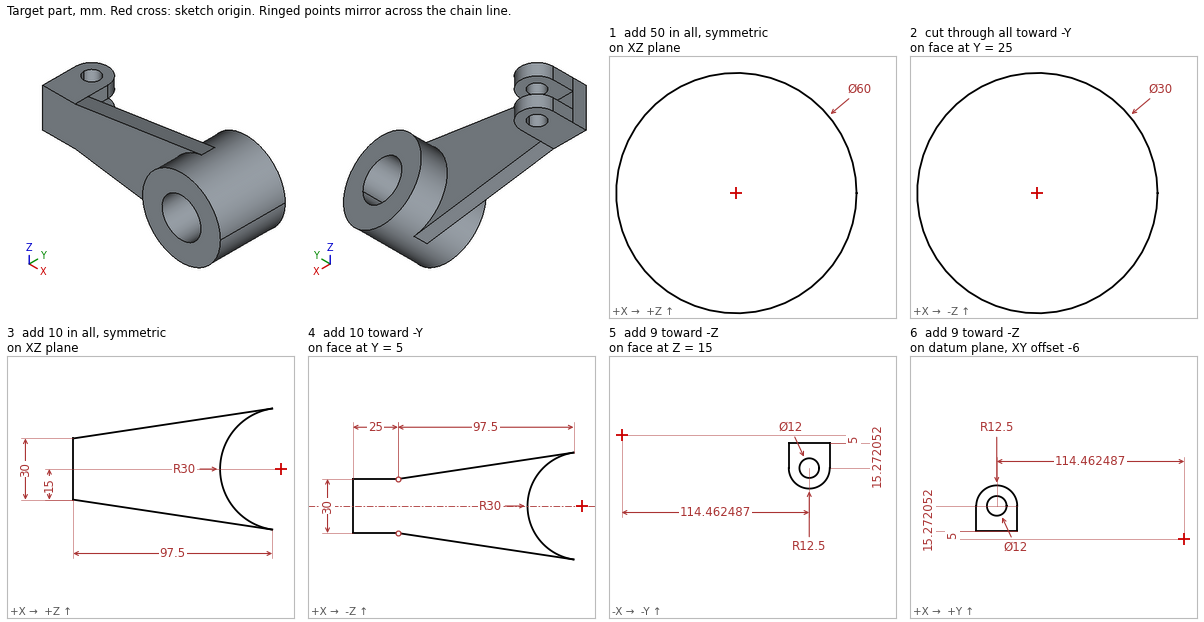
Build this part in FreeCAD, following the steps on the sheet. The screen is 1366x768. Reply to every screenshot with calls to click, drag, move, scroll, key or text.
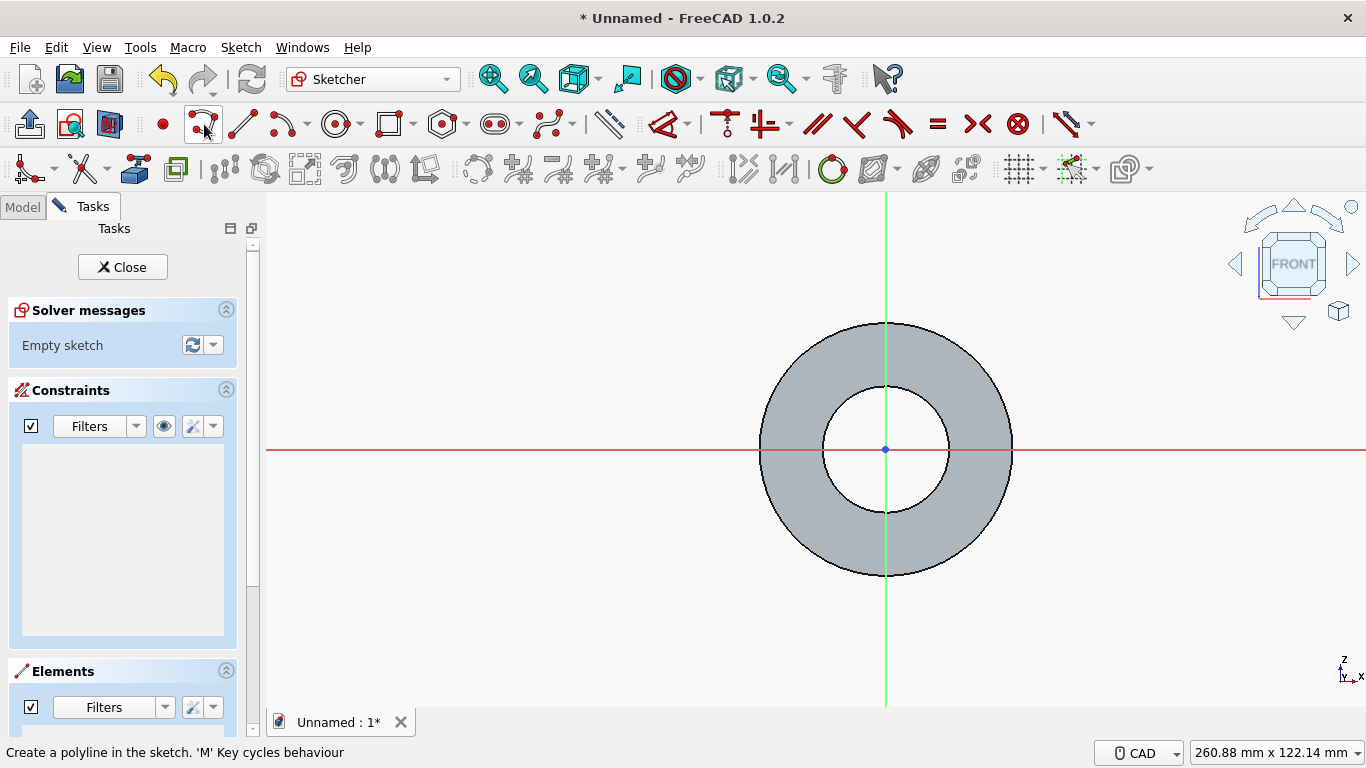
click(867, 575)
click(456, 513)
click(456, 386)
click(867, 324)
right_click(867, 324)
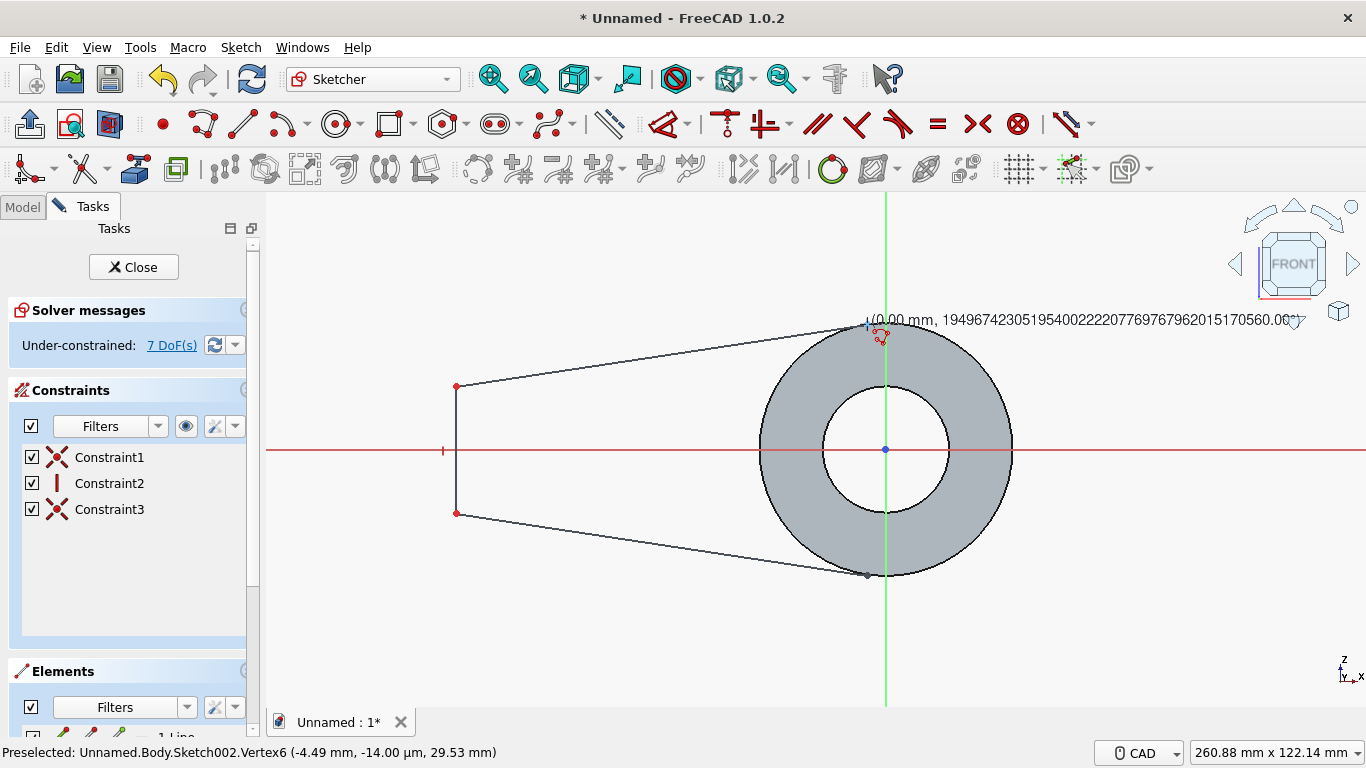
click(310, 124)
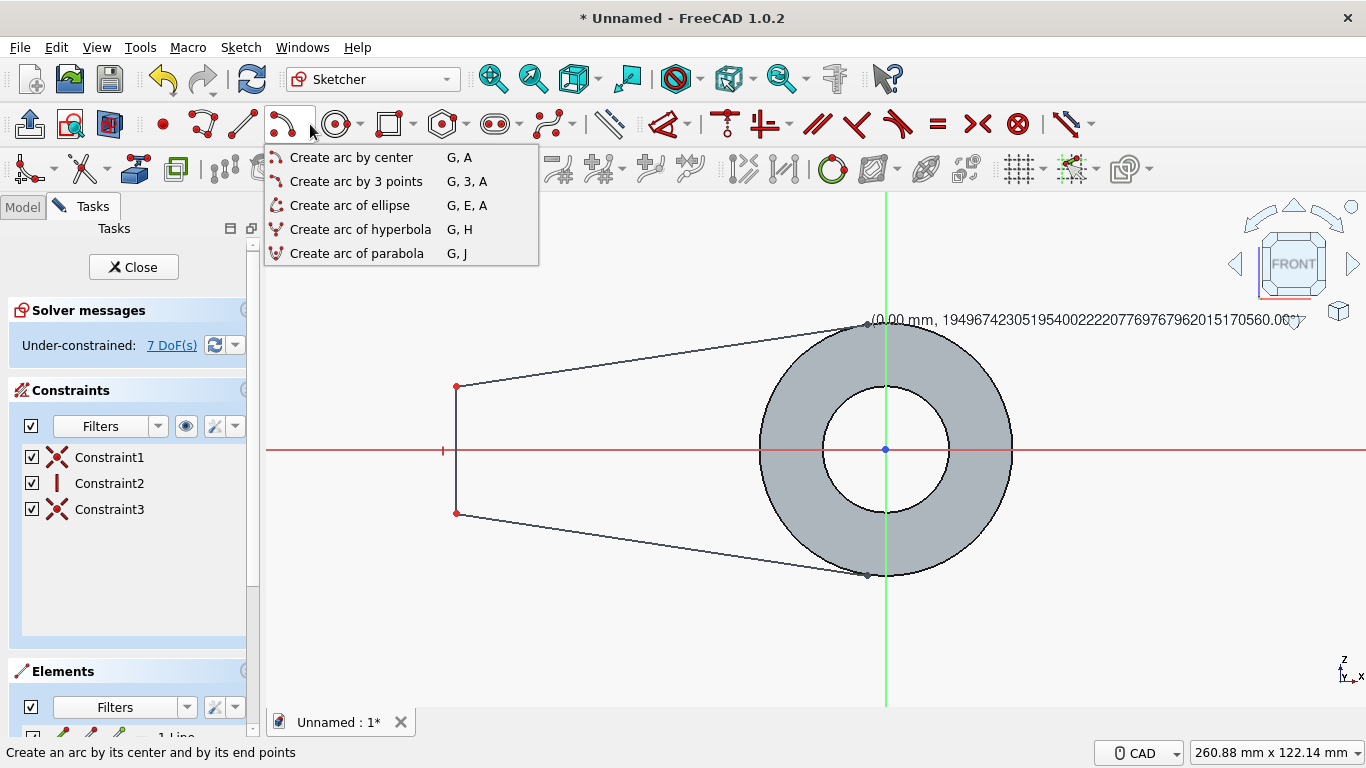
click(402, 181)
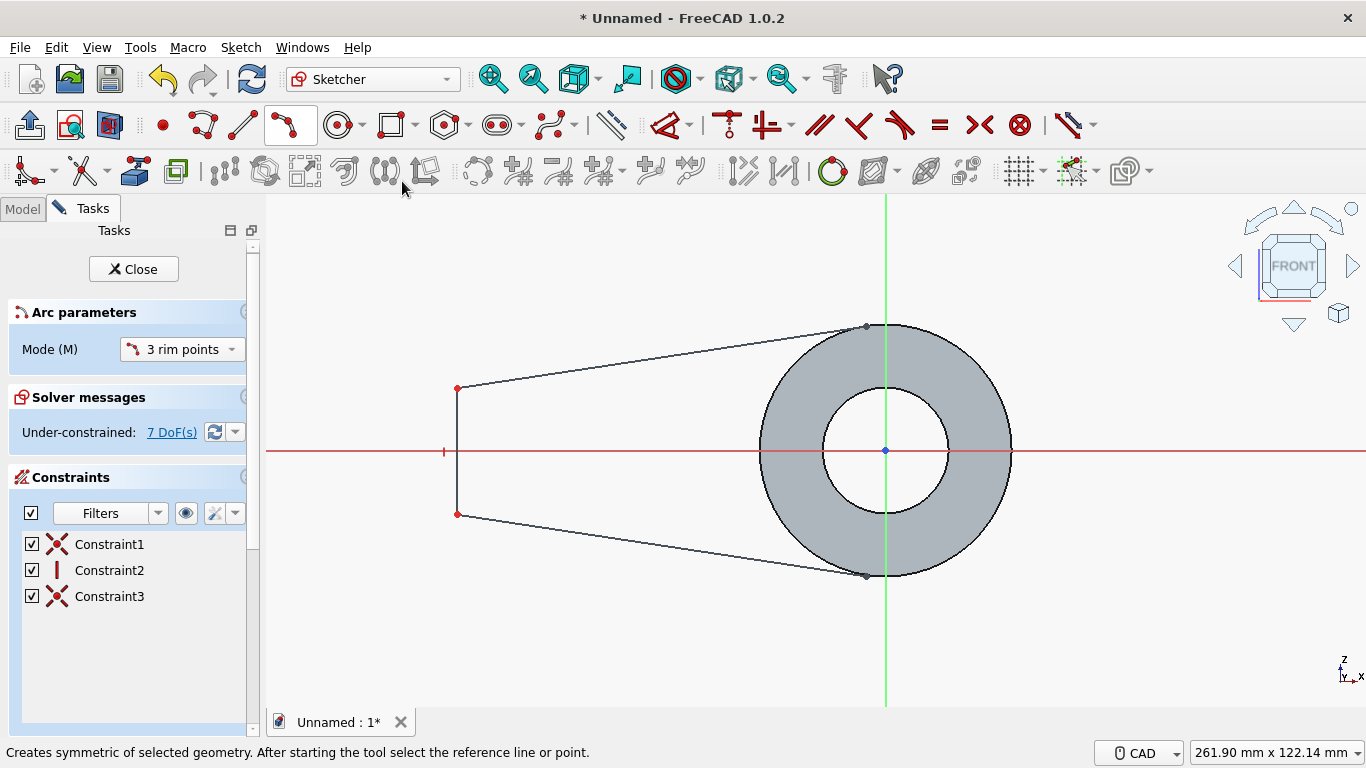
click(867, 326)
click(867, 577)
click(765, 415)
key(Escape)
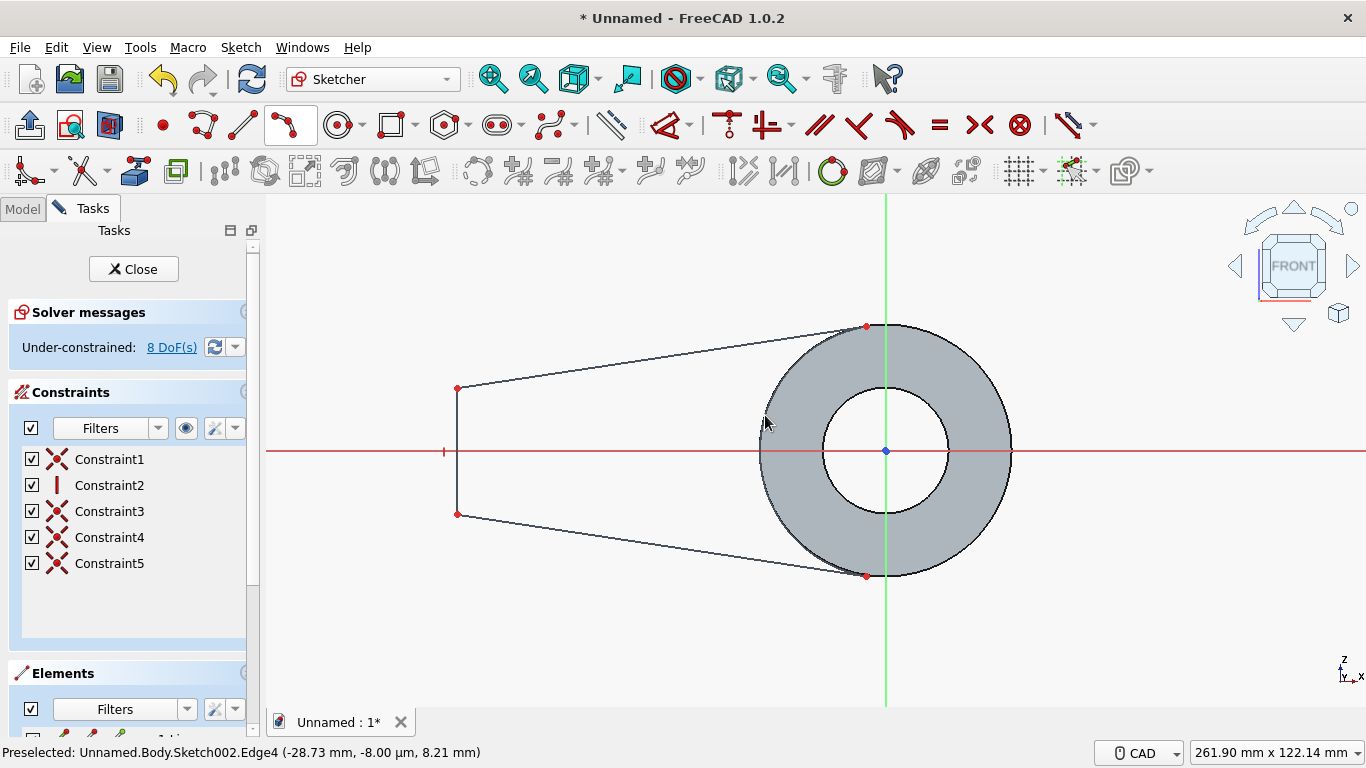
click(744, 558)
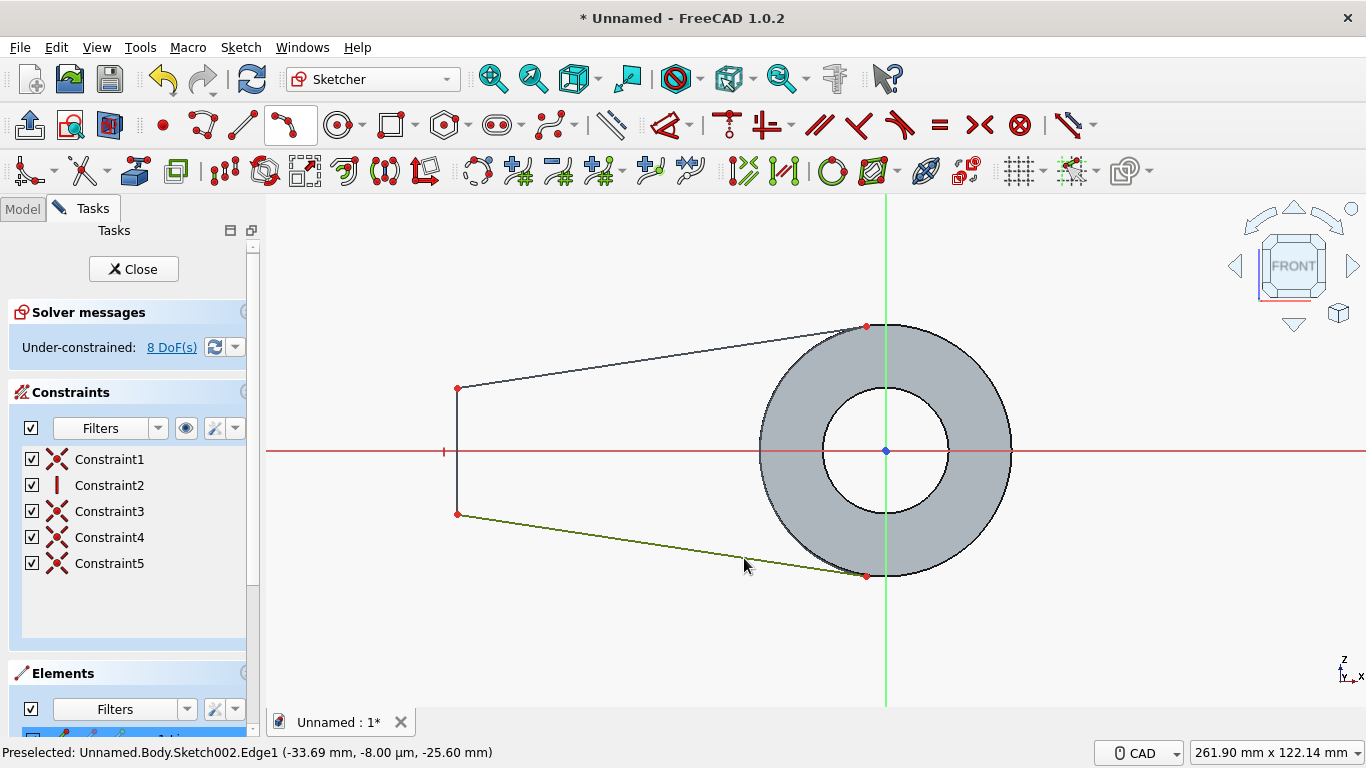
click(780, 384)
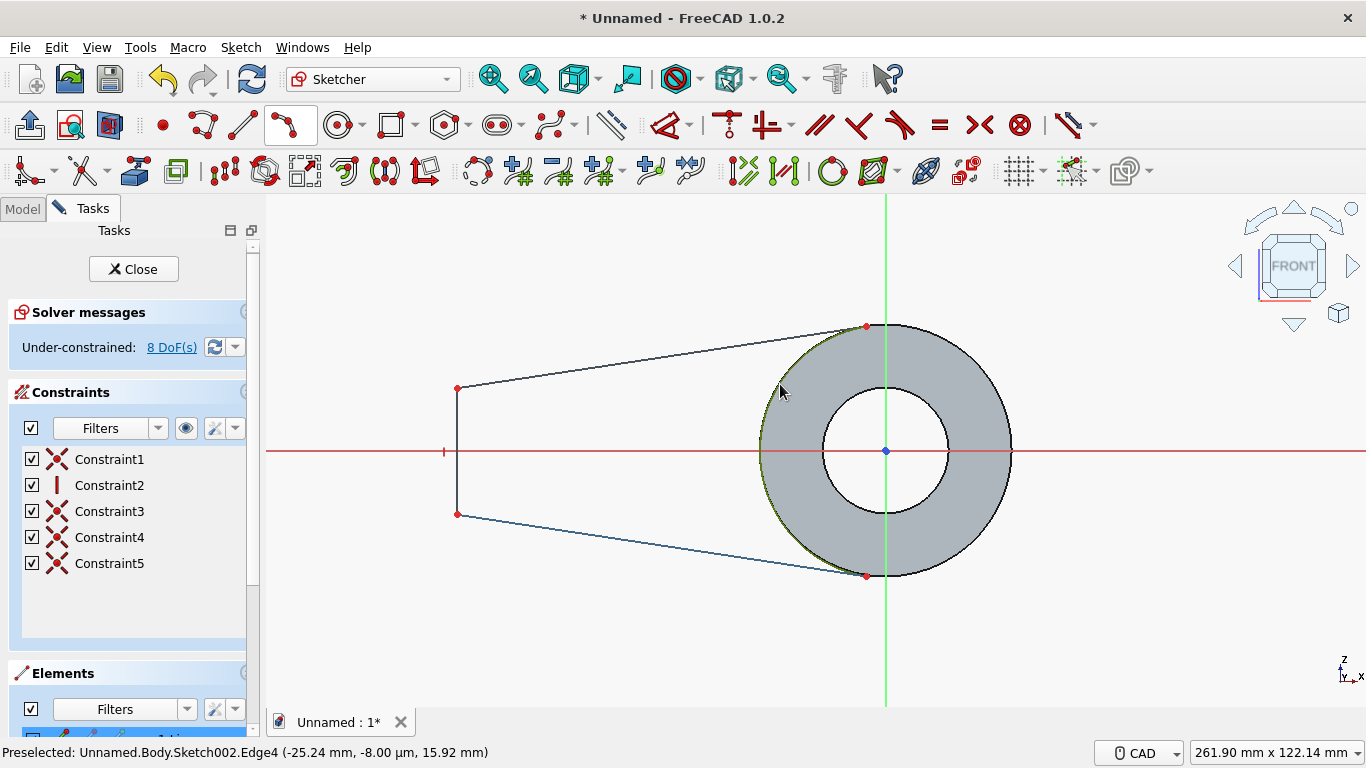
click(900, 126)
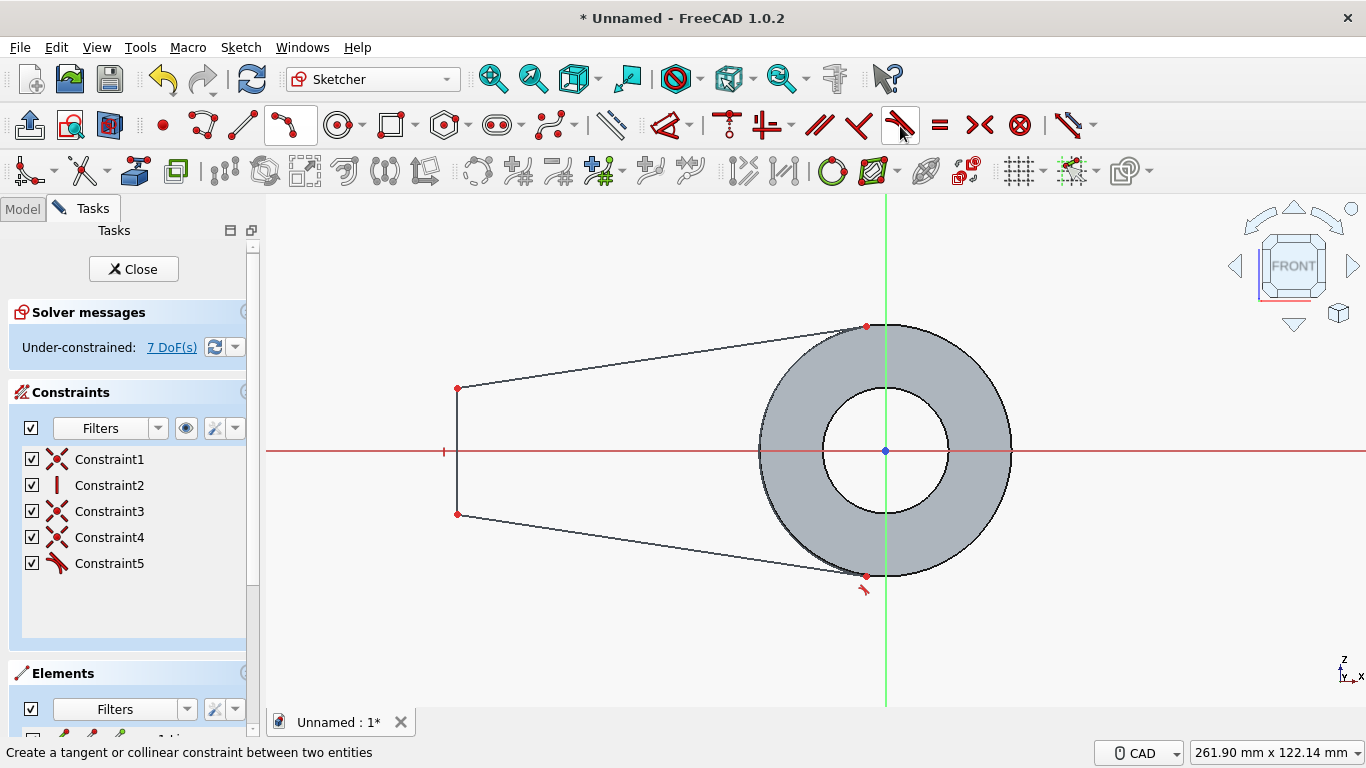
click(580, 370)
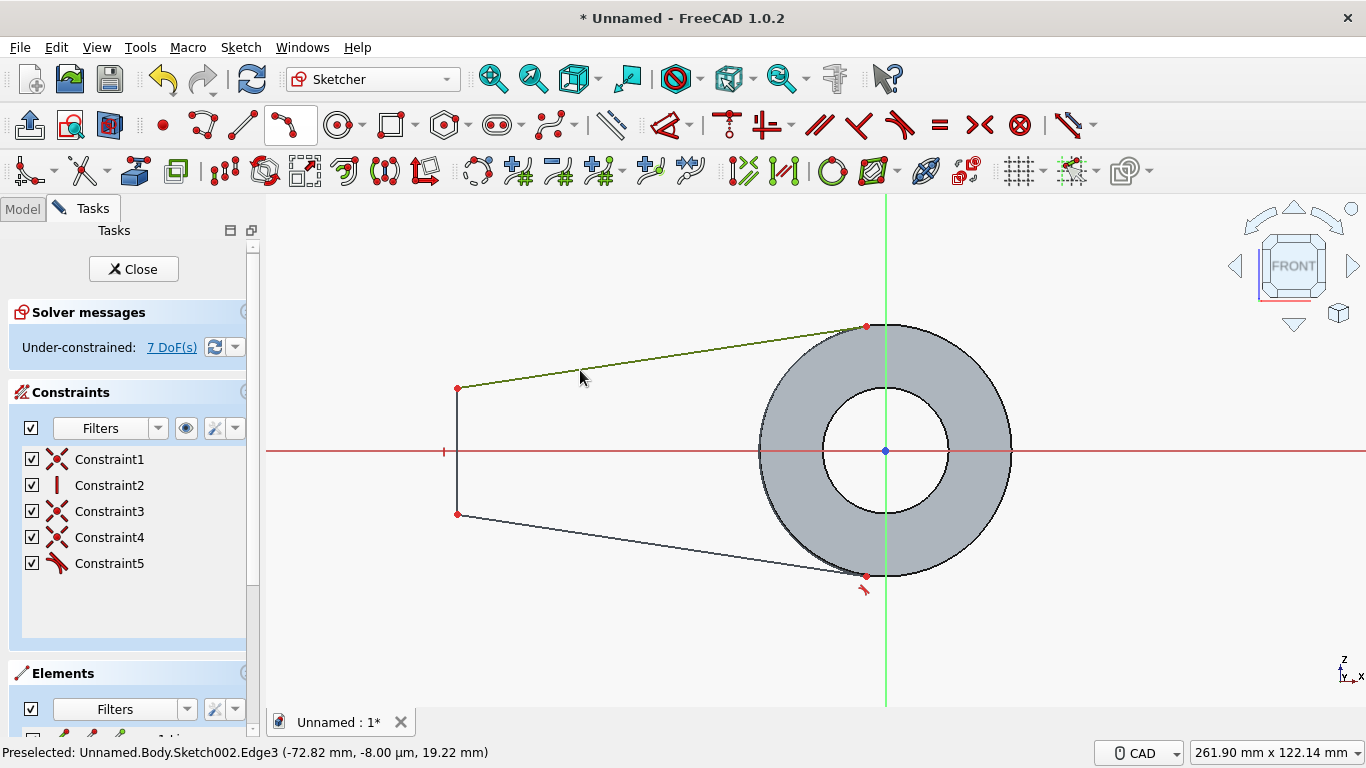
click(779, 383)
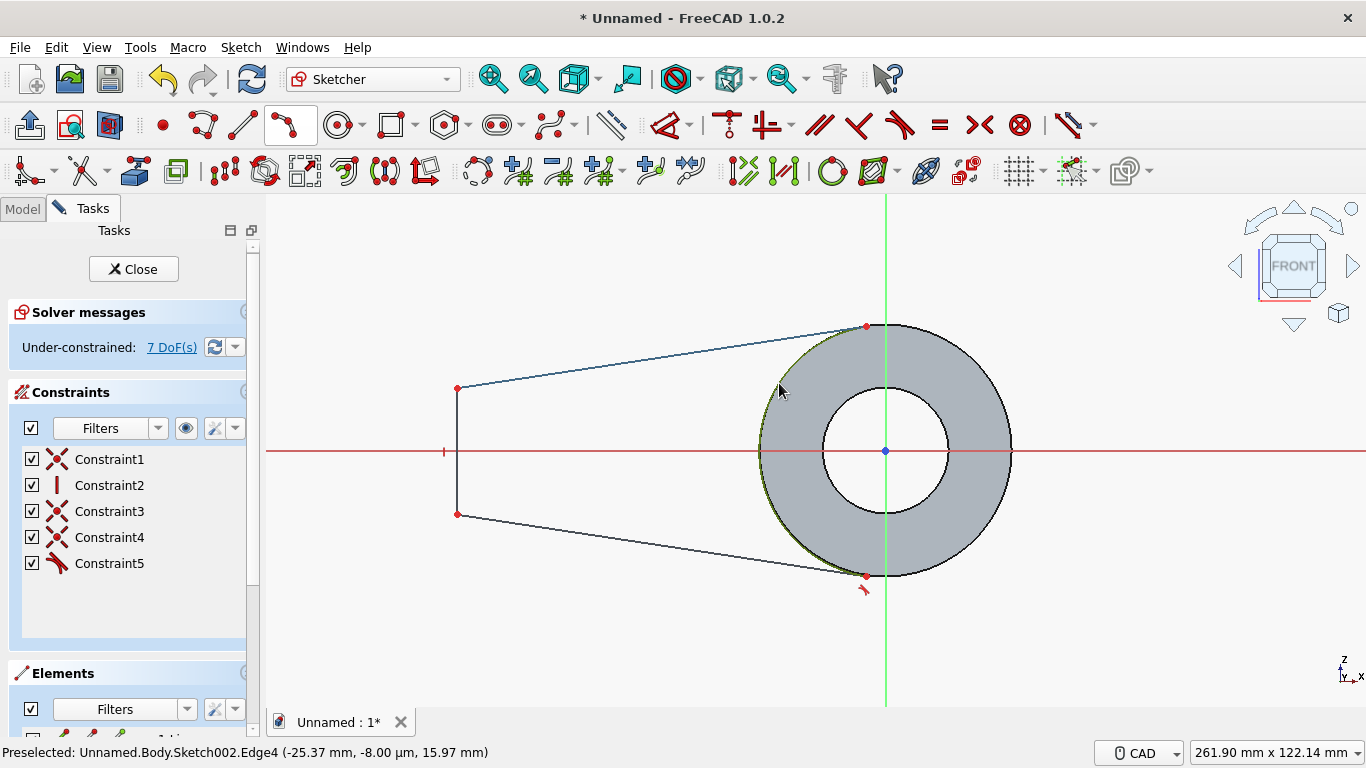
key(t)